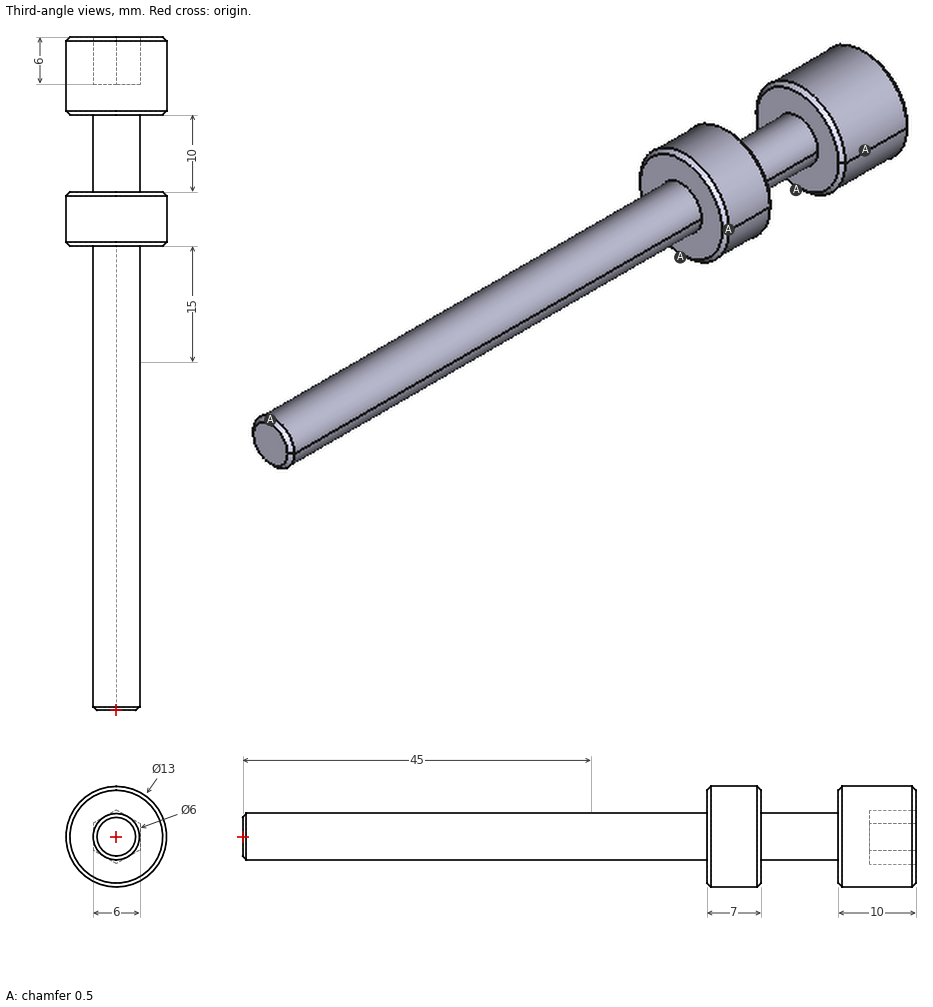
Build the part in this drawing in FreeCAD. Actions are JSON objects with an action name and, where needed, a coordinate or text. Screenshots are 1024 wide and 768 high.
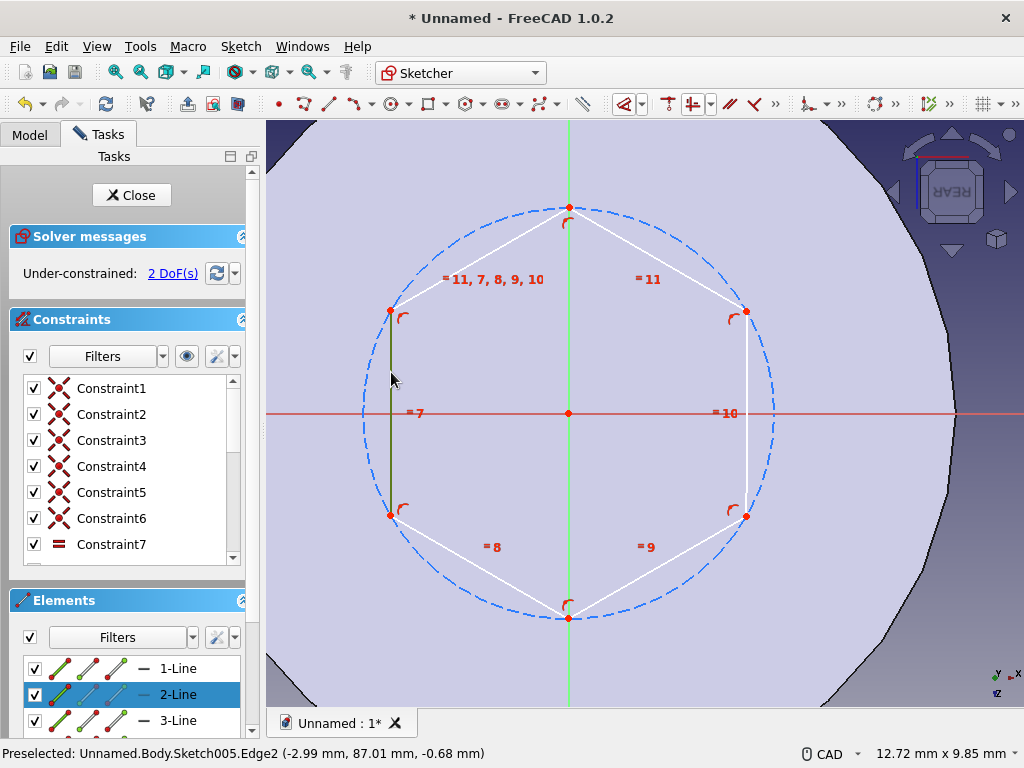
{"action": "key", "text": "v"}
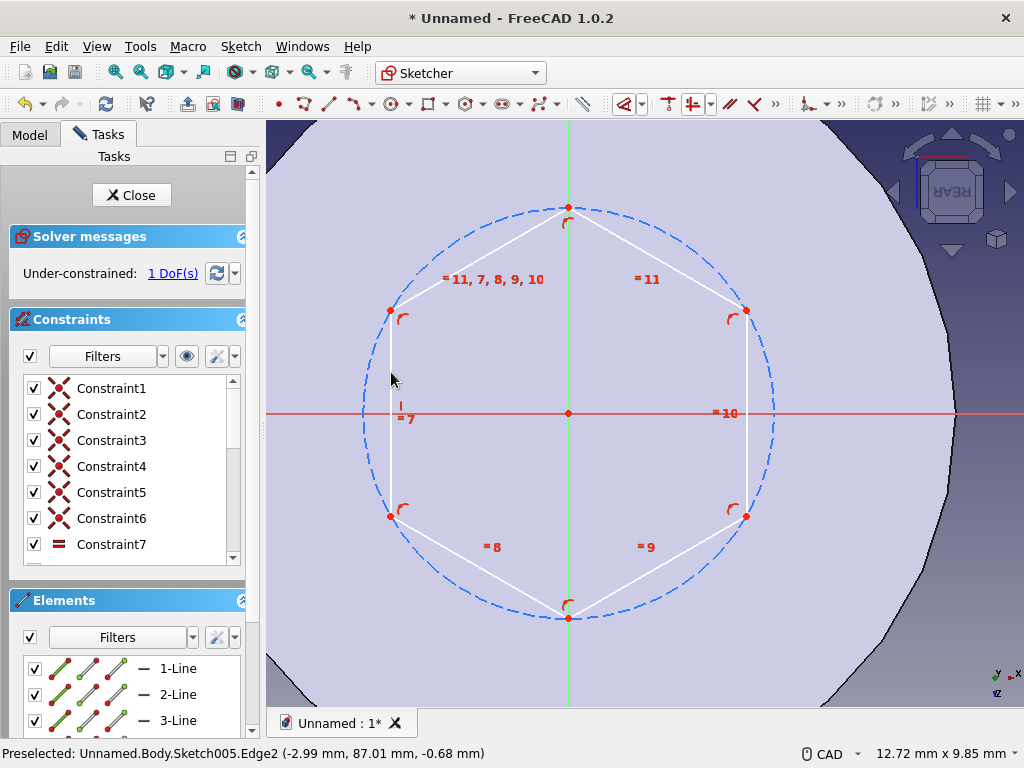
{"action": "left_click", "coordinate": [391, 311]}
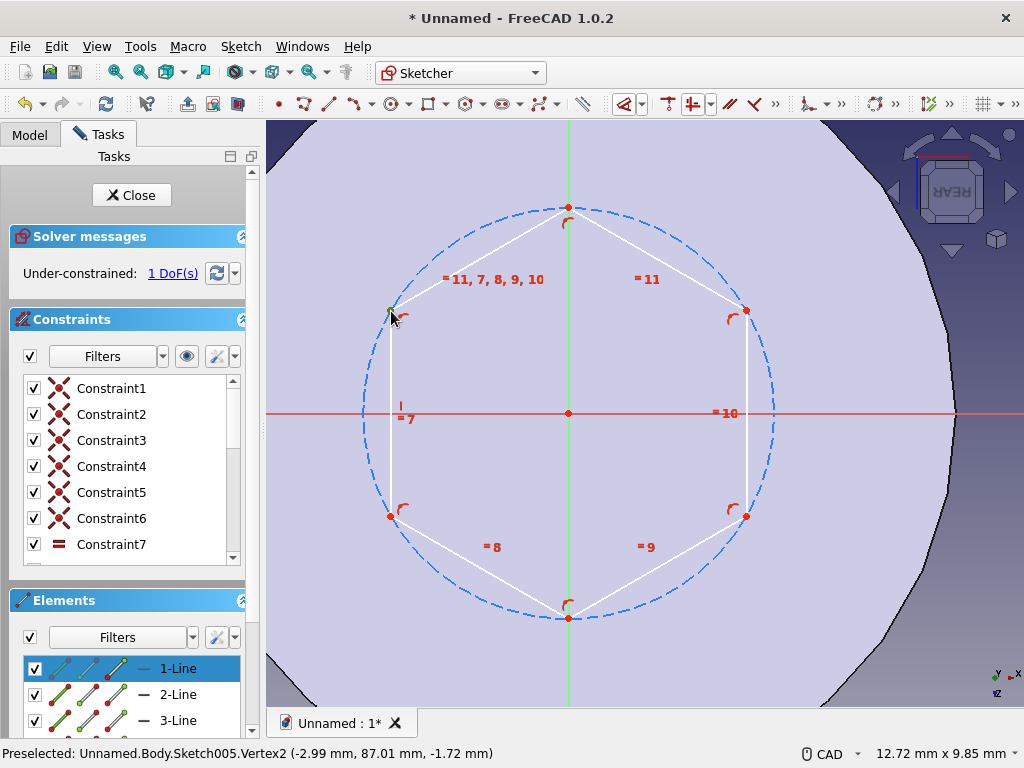
{"action": "left_click", "coordinate": [747, 516]}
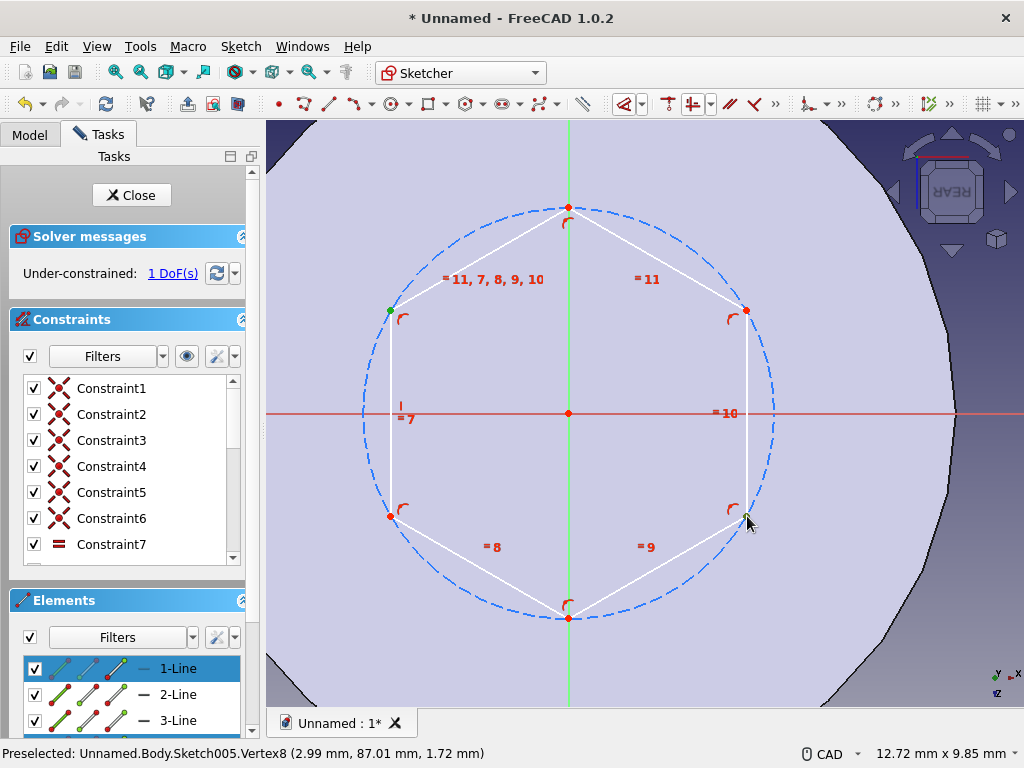
{"action": "key", "text": "l"}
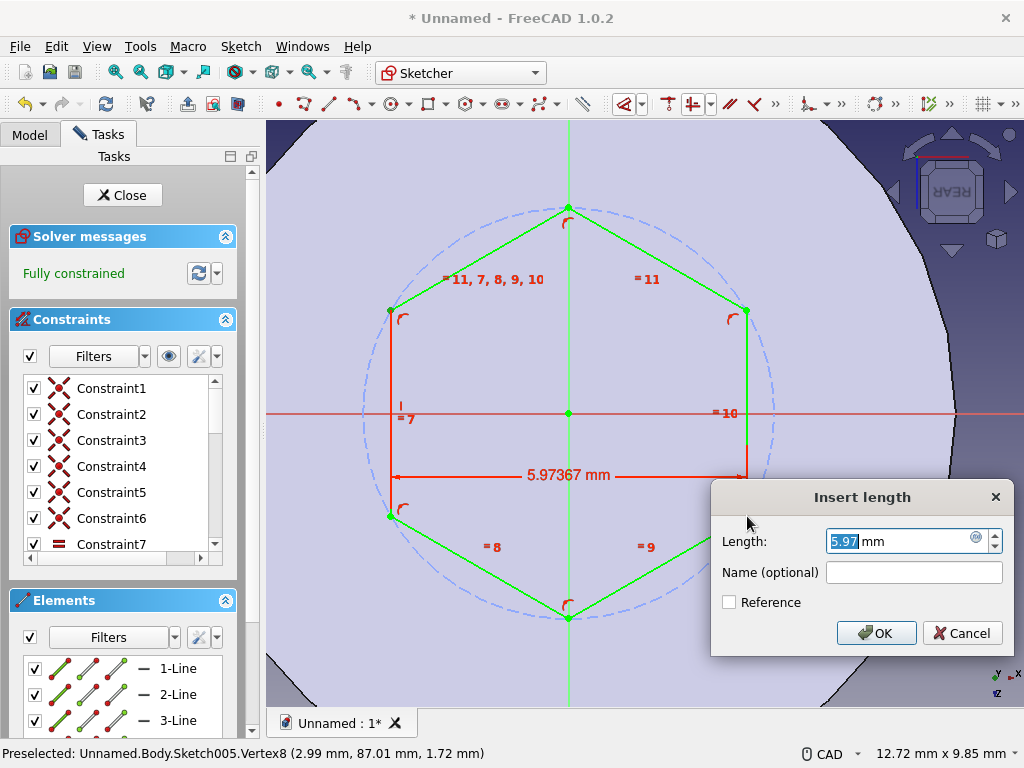
{"action": "type", "text": "6"}
{"action": "key", "text": "Return"}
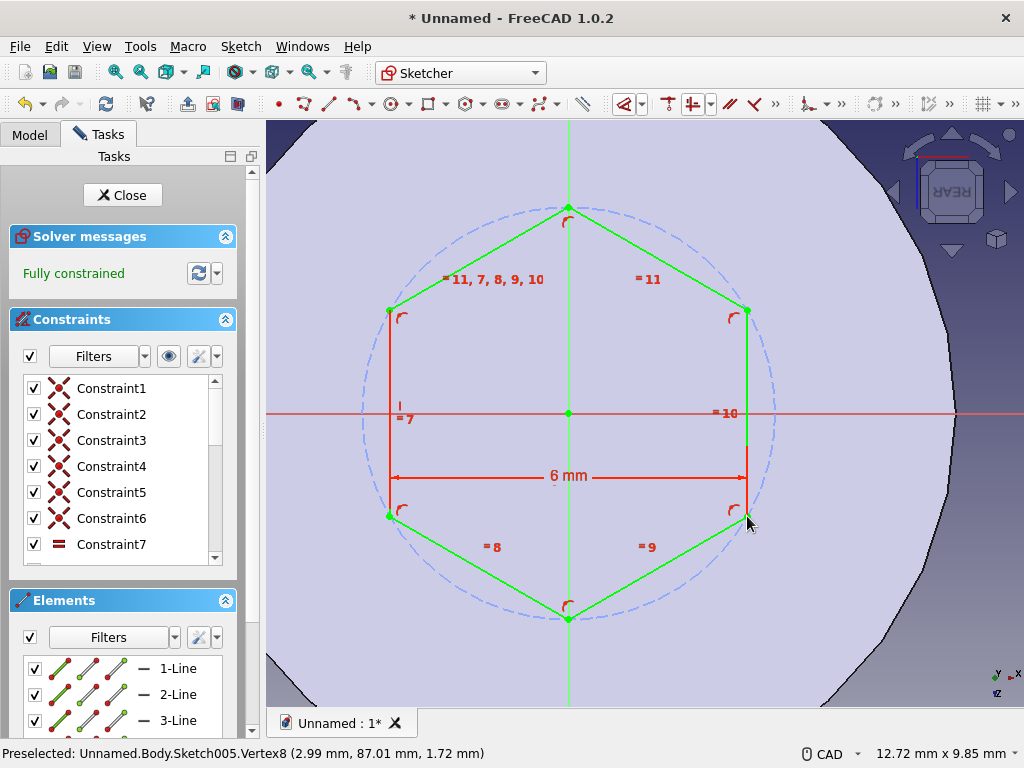
{"action": "left_click", "coordinate": [123, 195]}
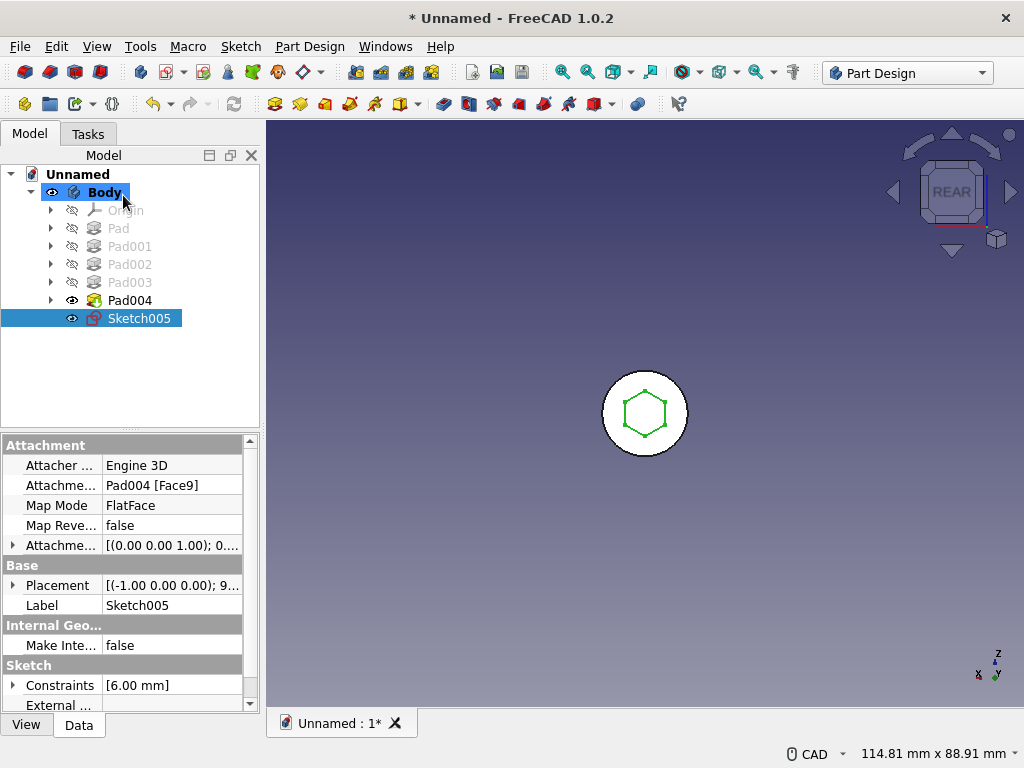
{"action": "left_click", "coordinate": [444, 104]}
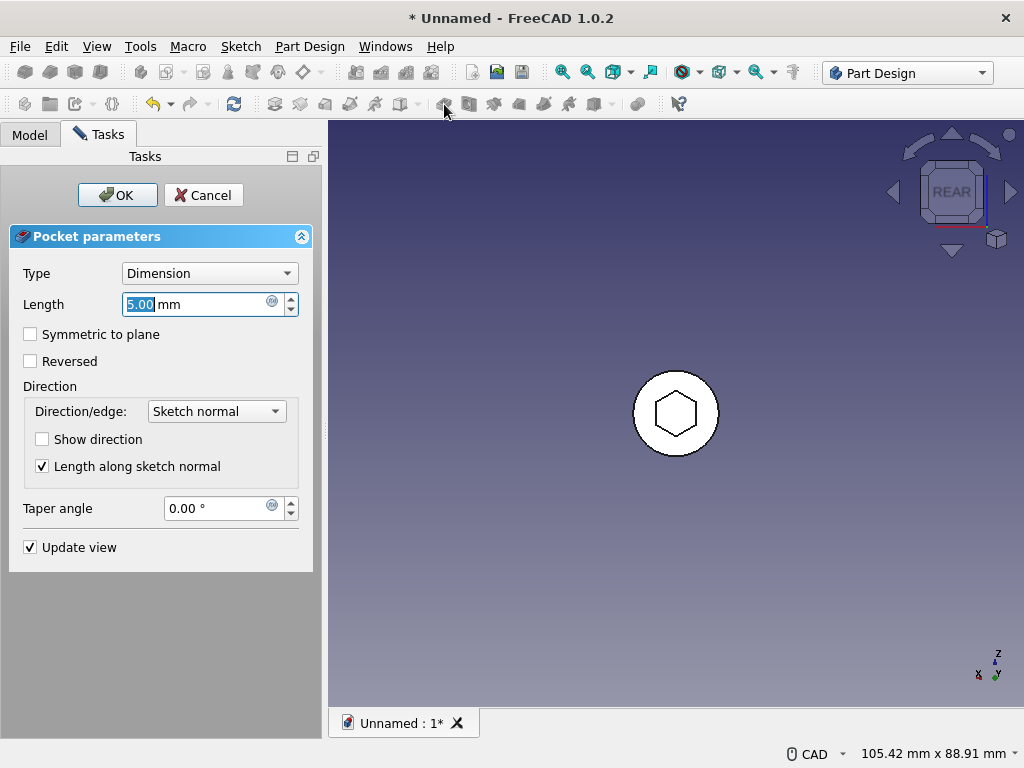
{"action": "type", "text": "6"}
{"action": "key", "text": "Tab"}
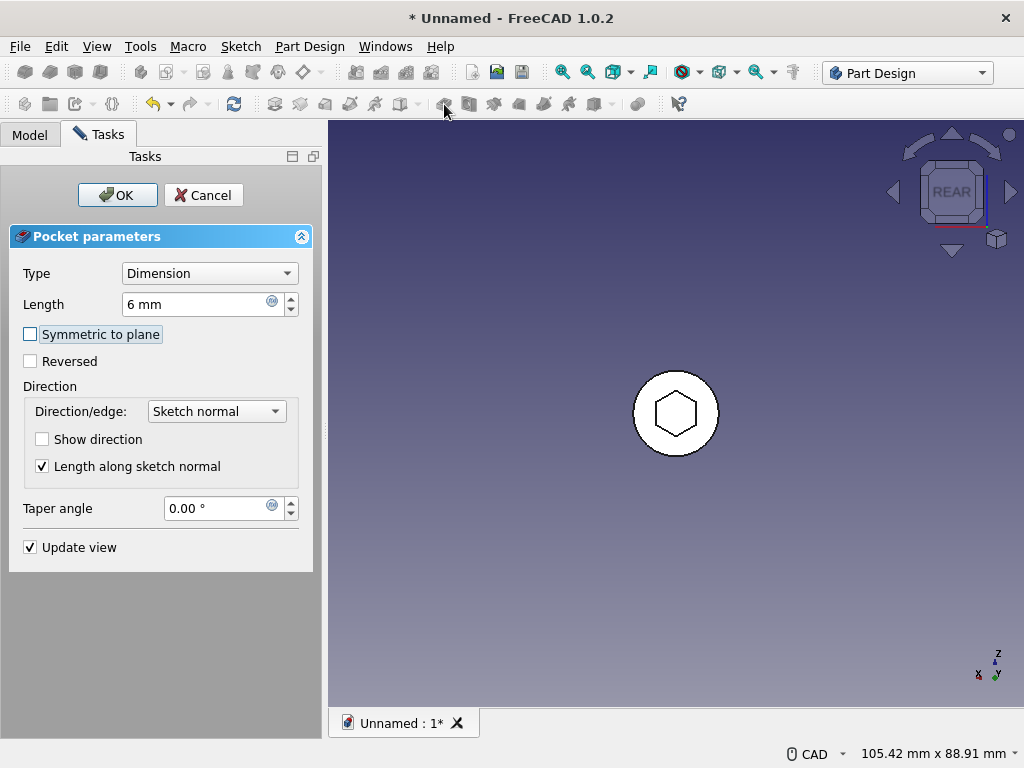
{"action": "left_click", "coordinate": [118, 195]}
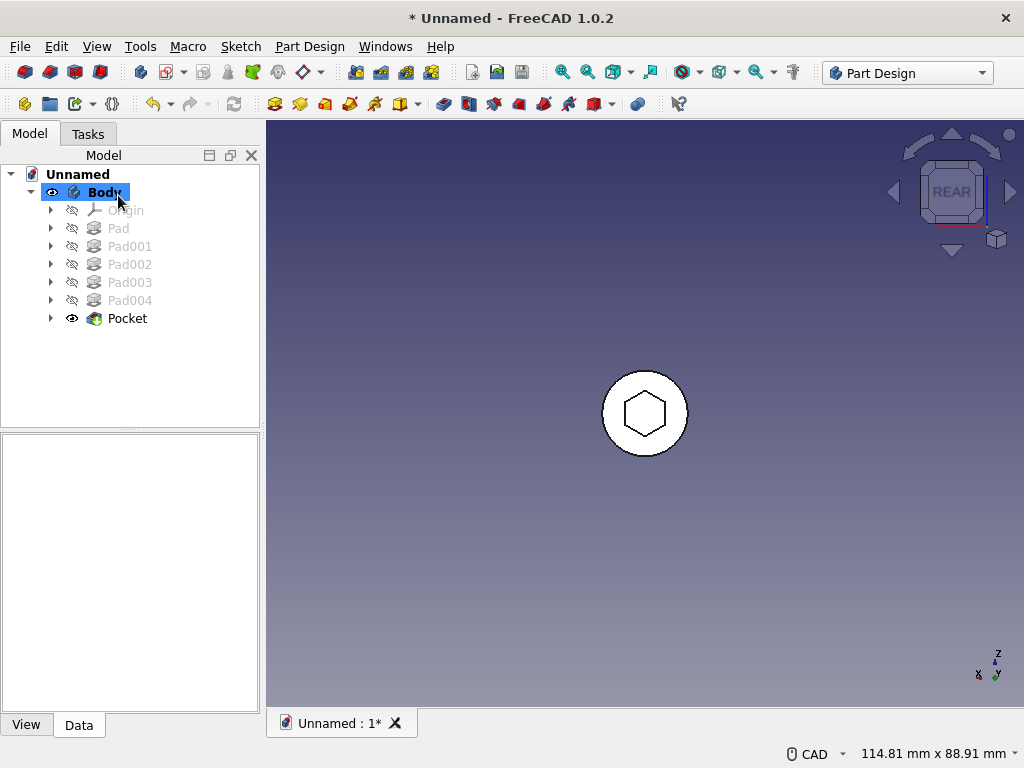
{"action": "left_click", "coordinate": [563, 72]}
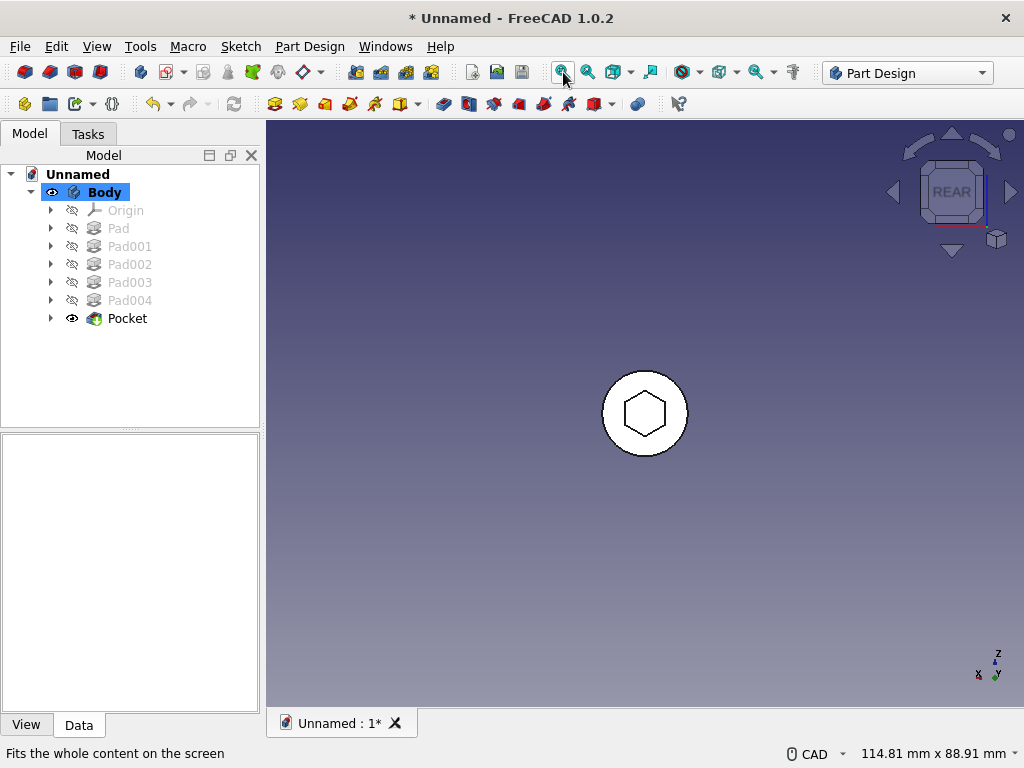
{"action": "left_click", "coordinate": [688, 412]}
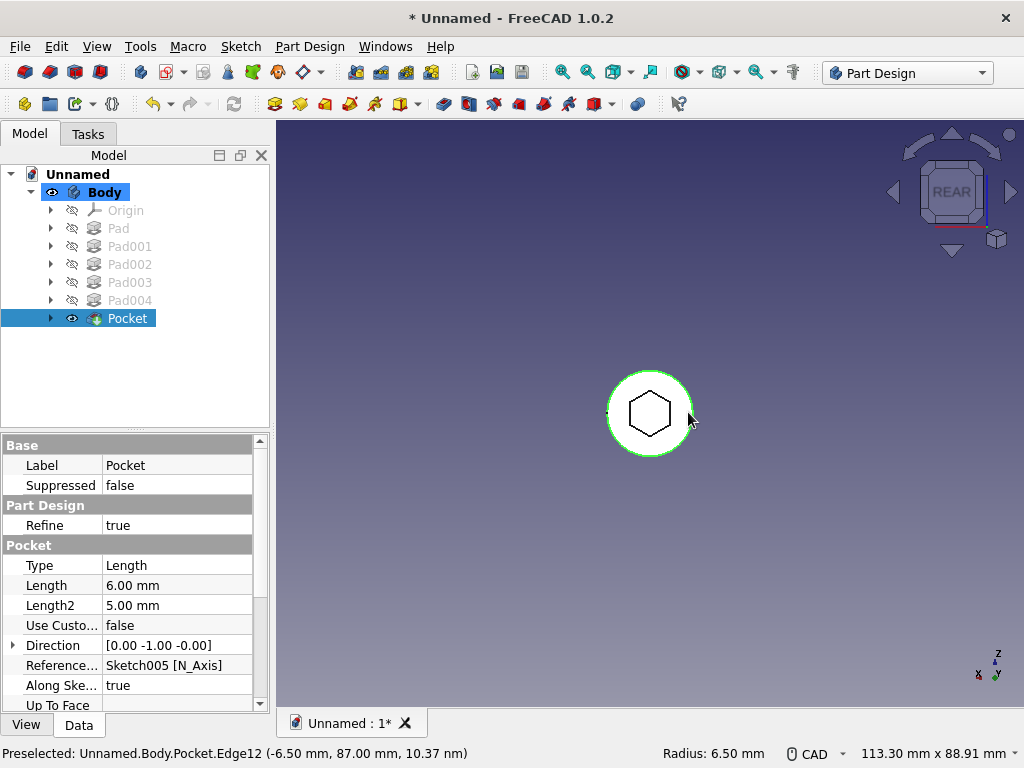
{"action": "key", "text": "0"}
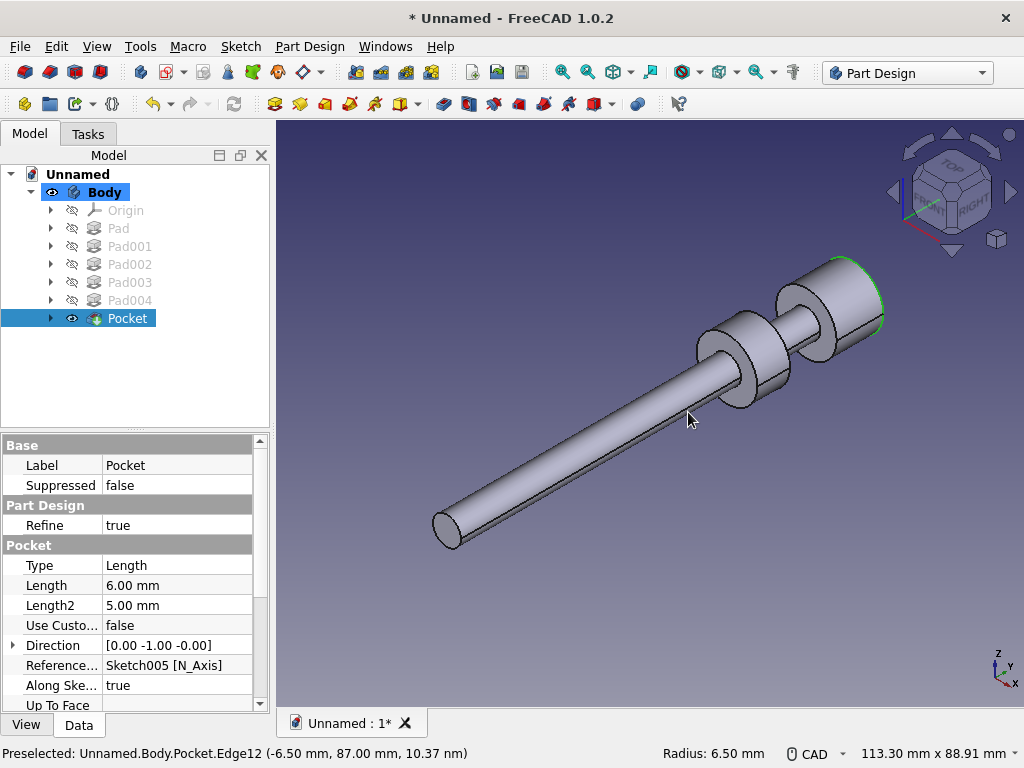
{"action": "left_click", "coordinate": [797, 283], "text": "ctrl"}